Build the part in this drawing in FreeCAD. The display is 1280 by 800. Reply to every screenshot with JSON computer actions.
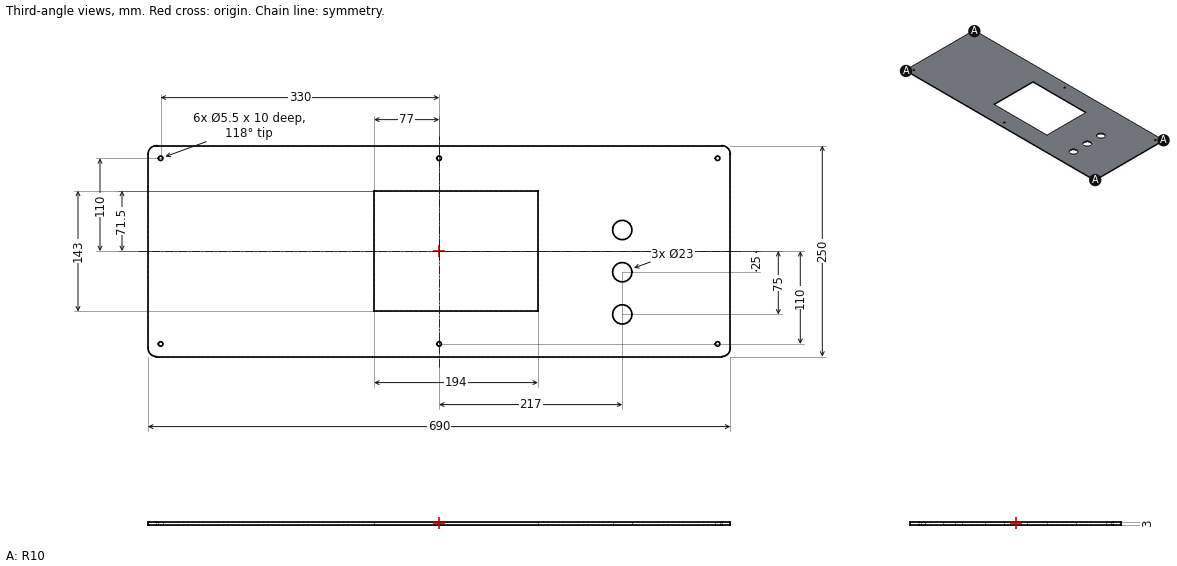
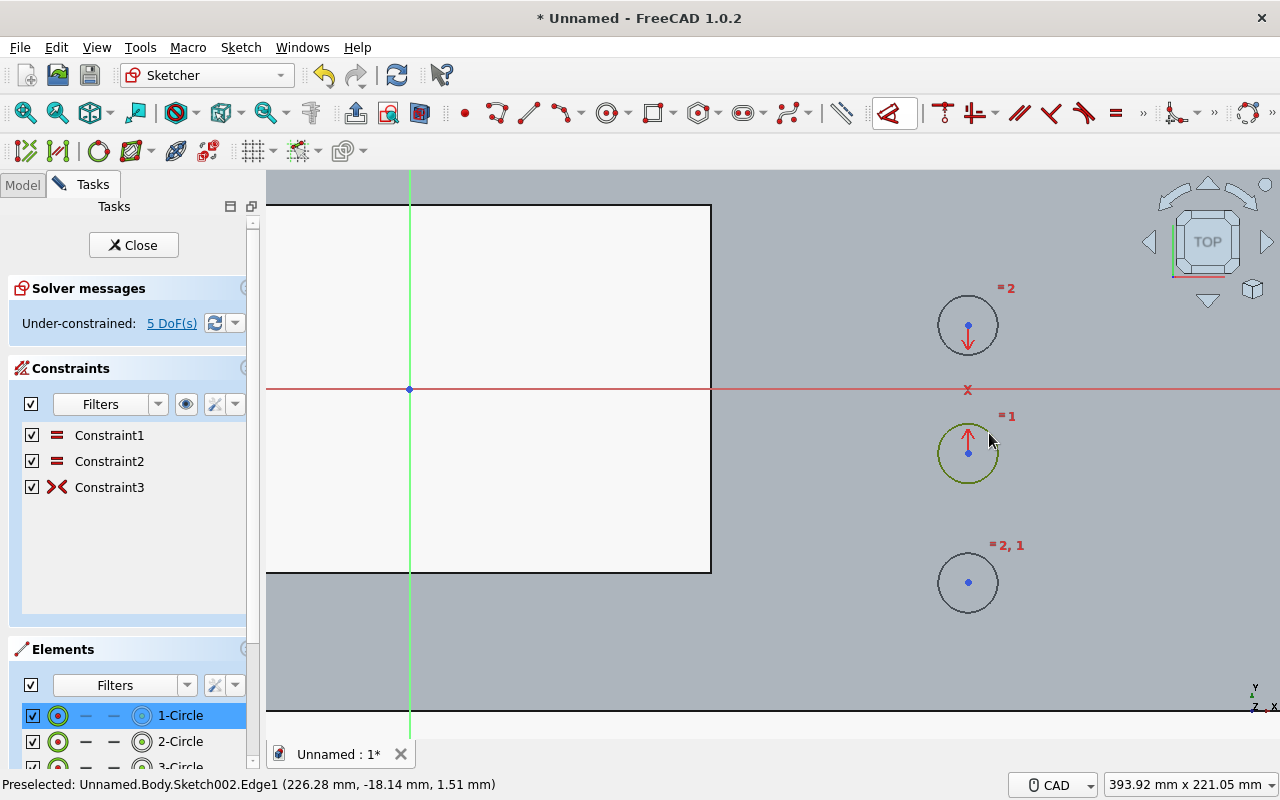
{"action": "left_click", "coordinate": [912, 114]}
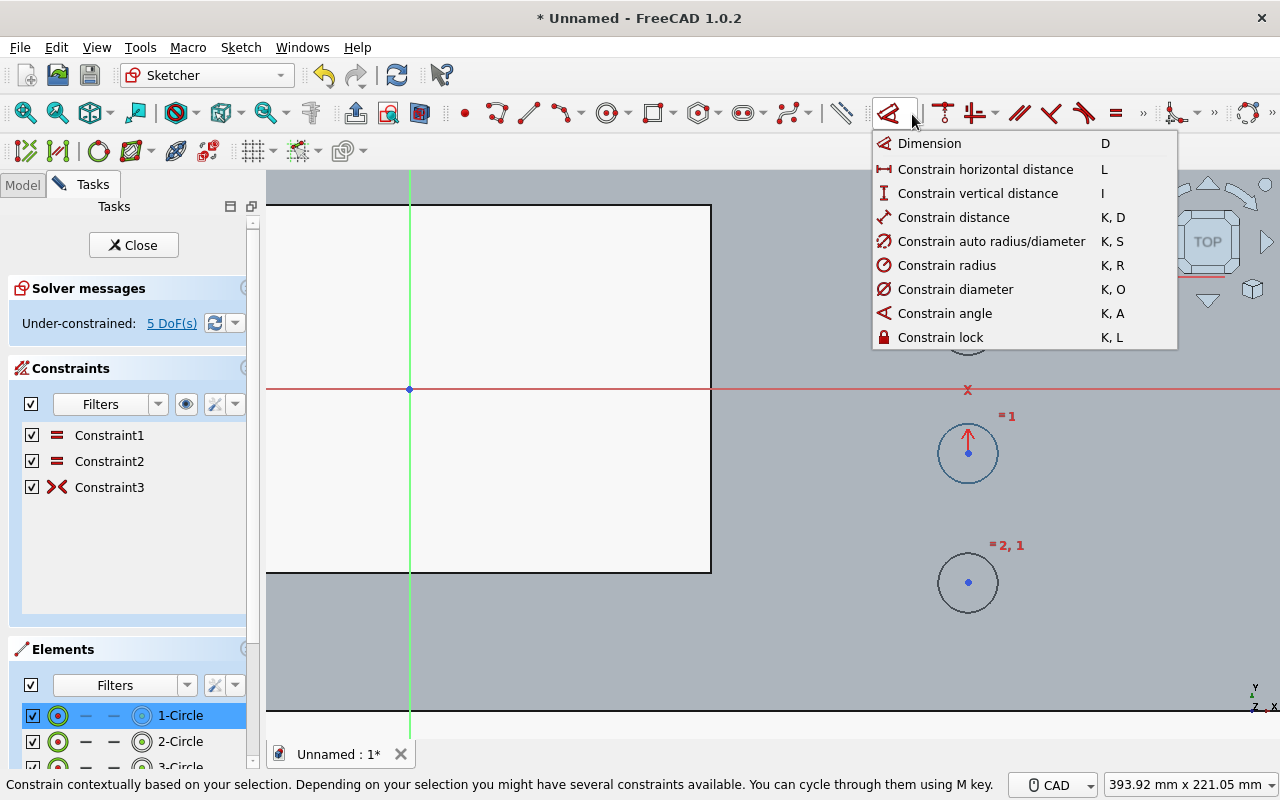
{"action": "left_click", "coordinate": [1025, 289]}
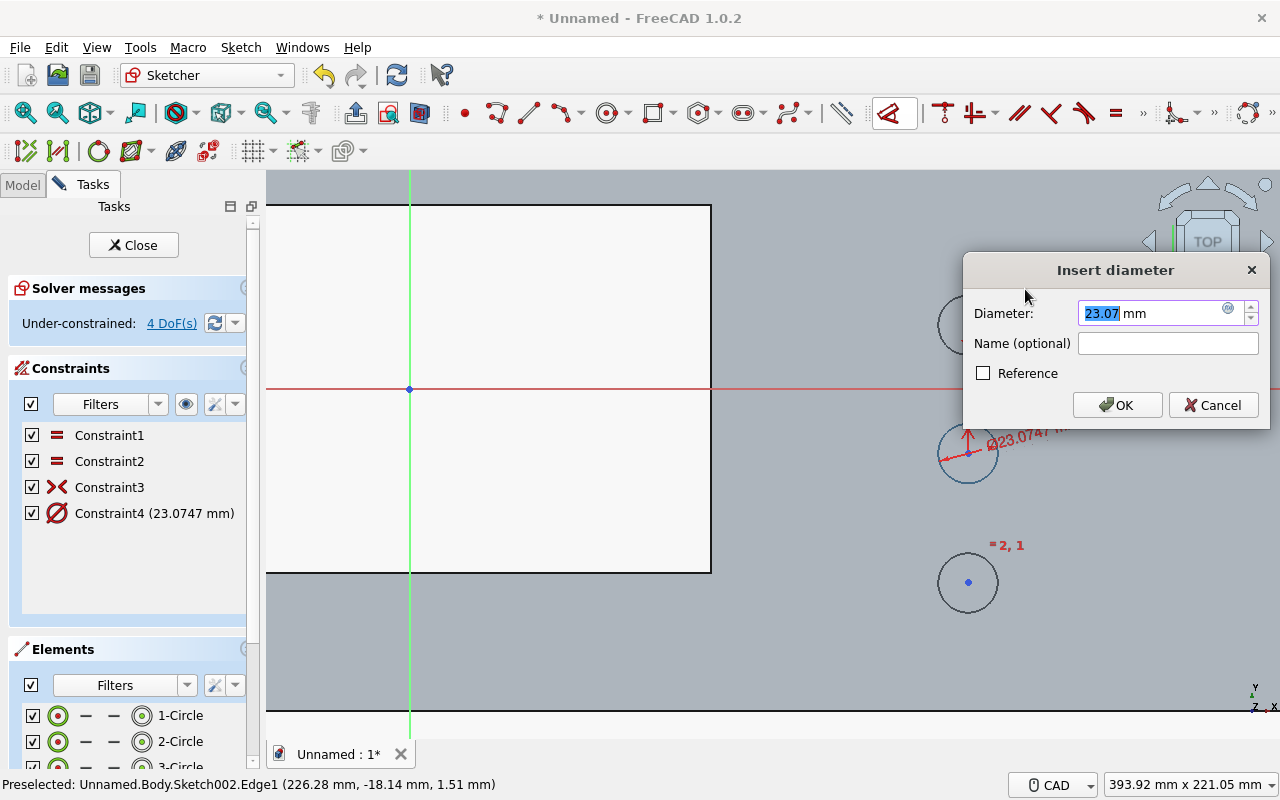
{"action": "type", "text": "23"}
{"action": "key", "text": "Return"}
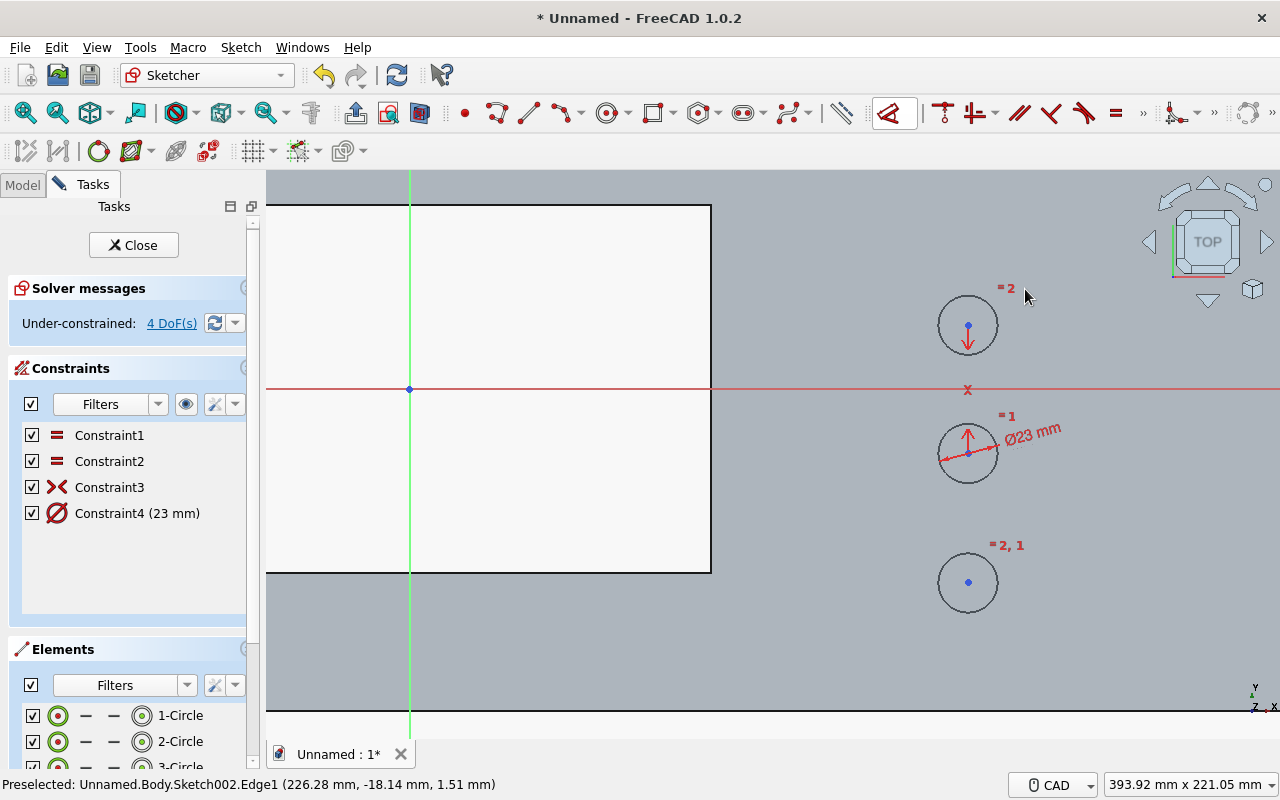
{"action": "left_click", "coordinate": [968, 454]}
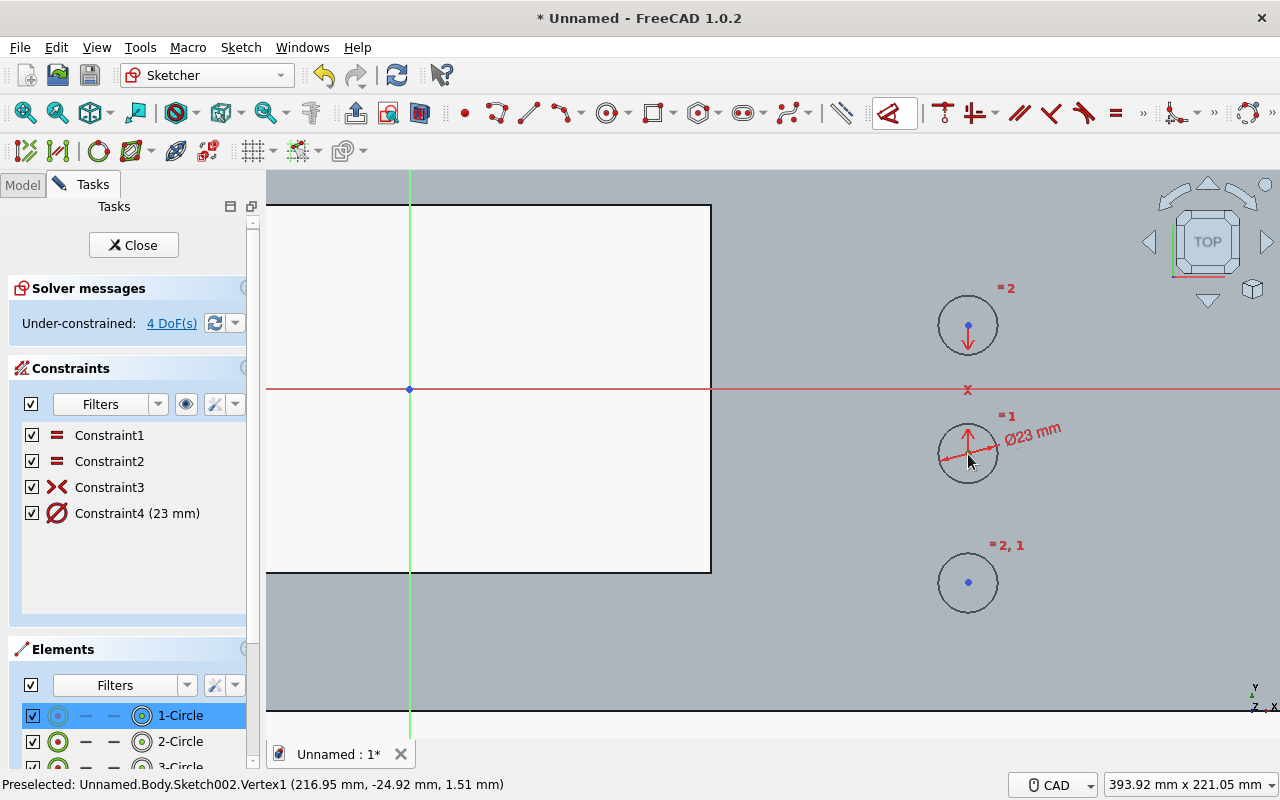
{"action": "left_click", "coordinate": [912, 114]}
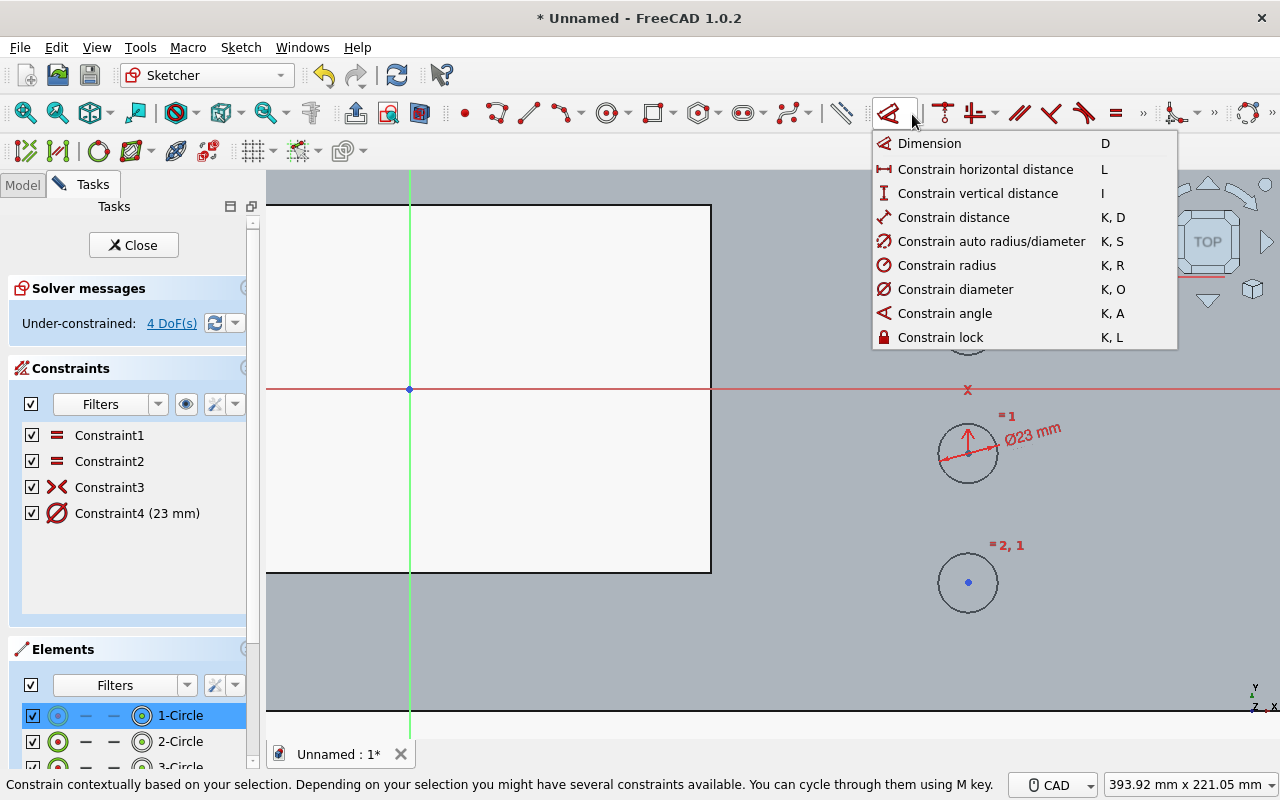
{"action": "left_click", "coordinate": [1025, 193]}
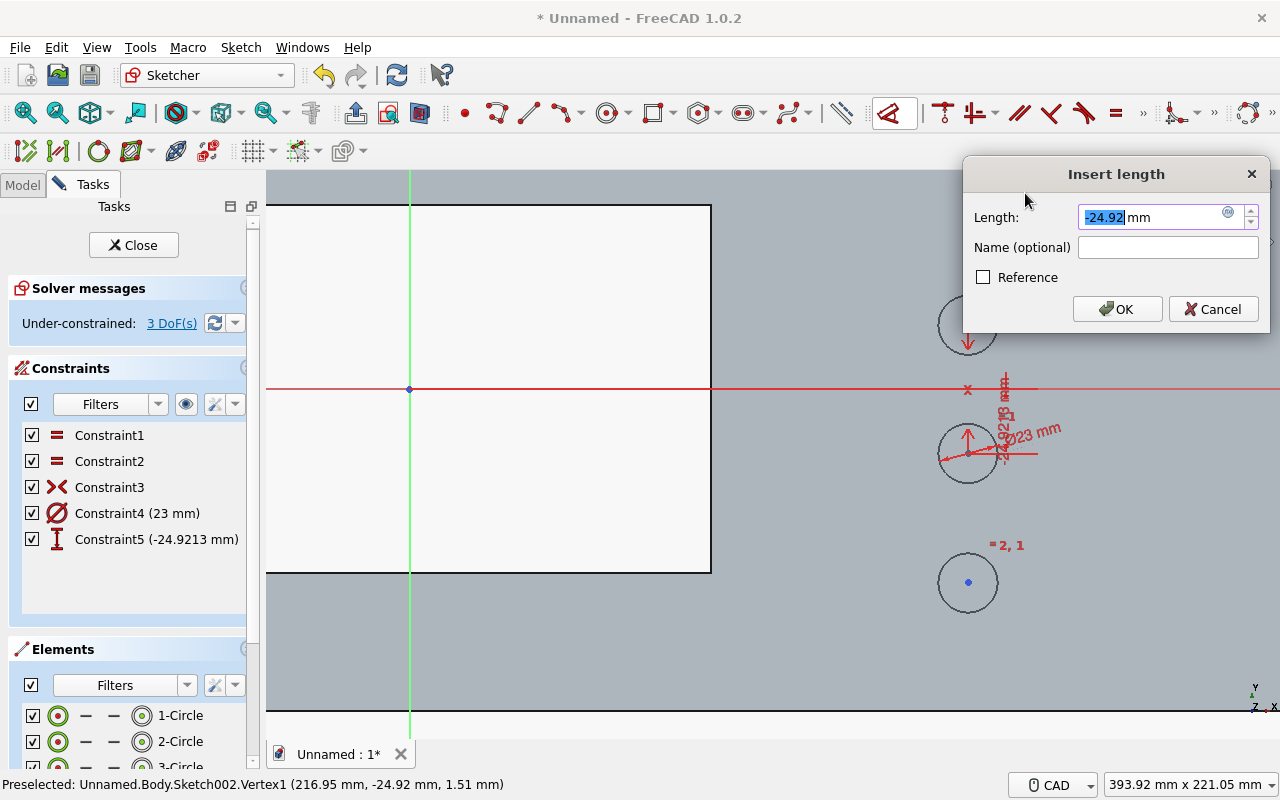
{"action": "type", "text": "-25"}
{"action": "key", "text": "Return"}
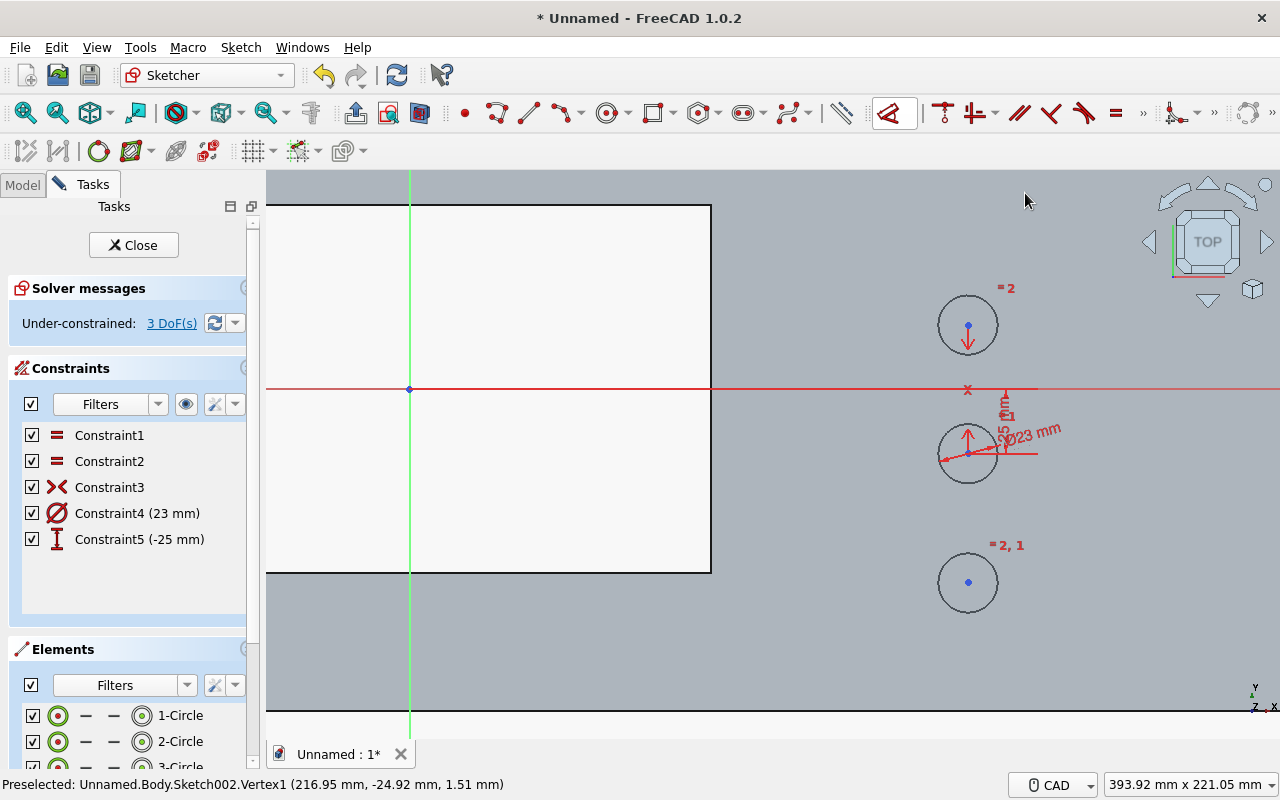
{"action": "left_click", "coordinate": [968, 583]}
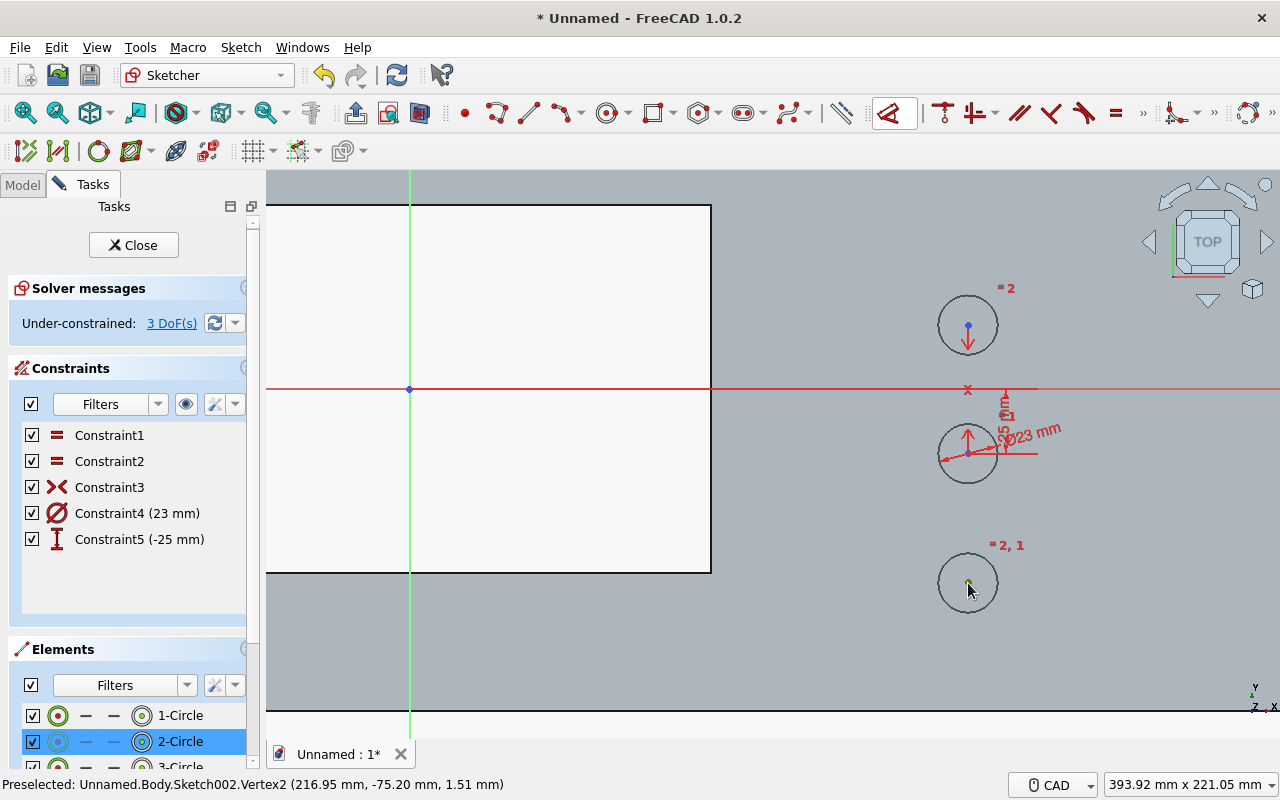
{"action": "key", "text": "i"}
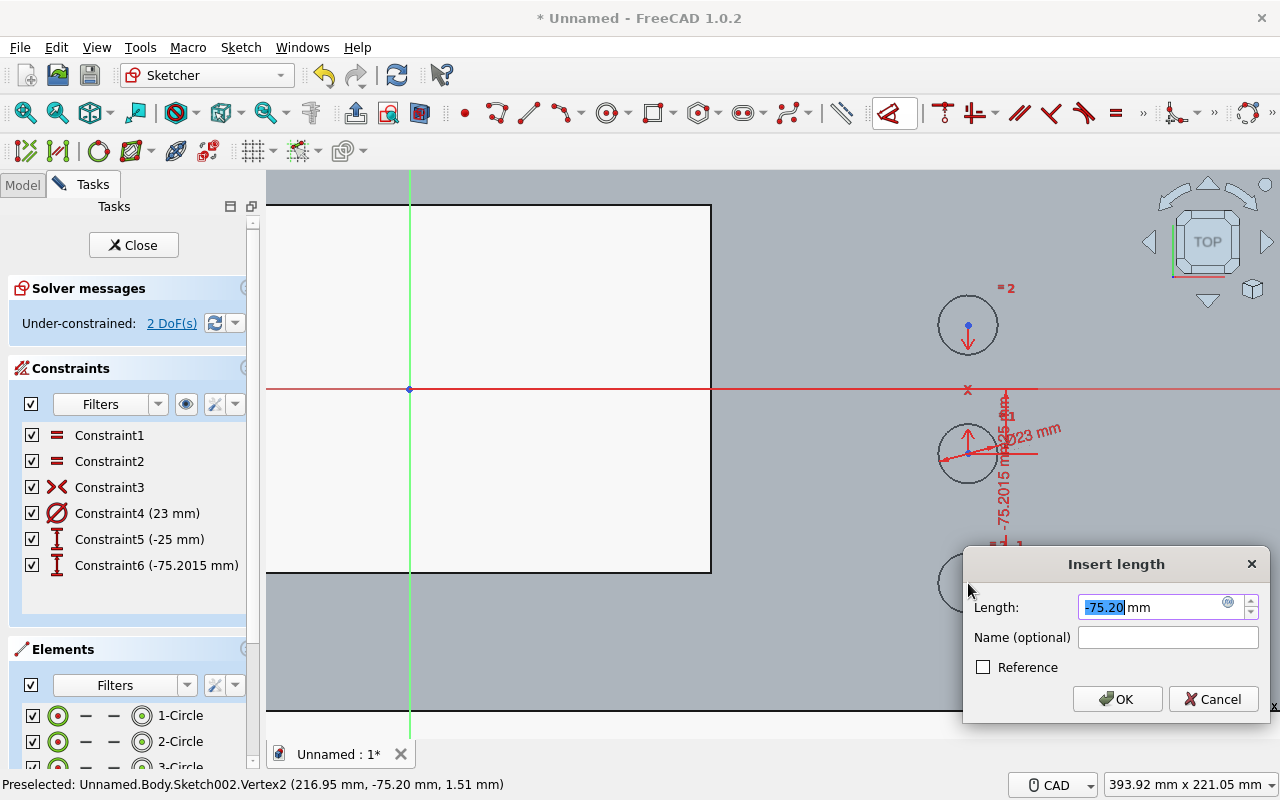
{"action": "type", "text": "-75"}
{"action": "key", "text": "Return"}